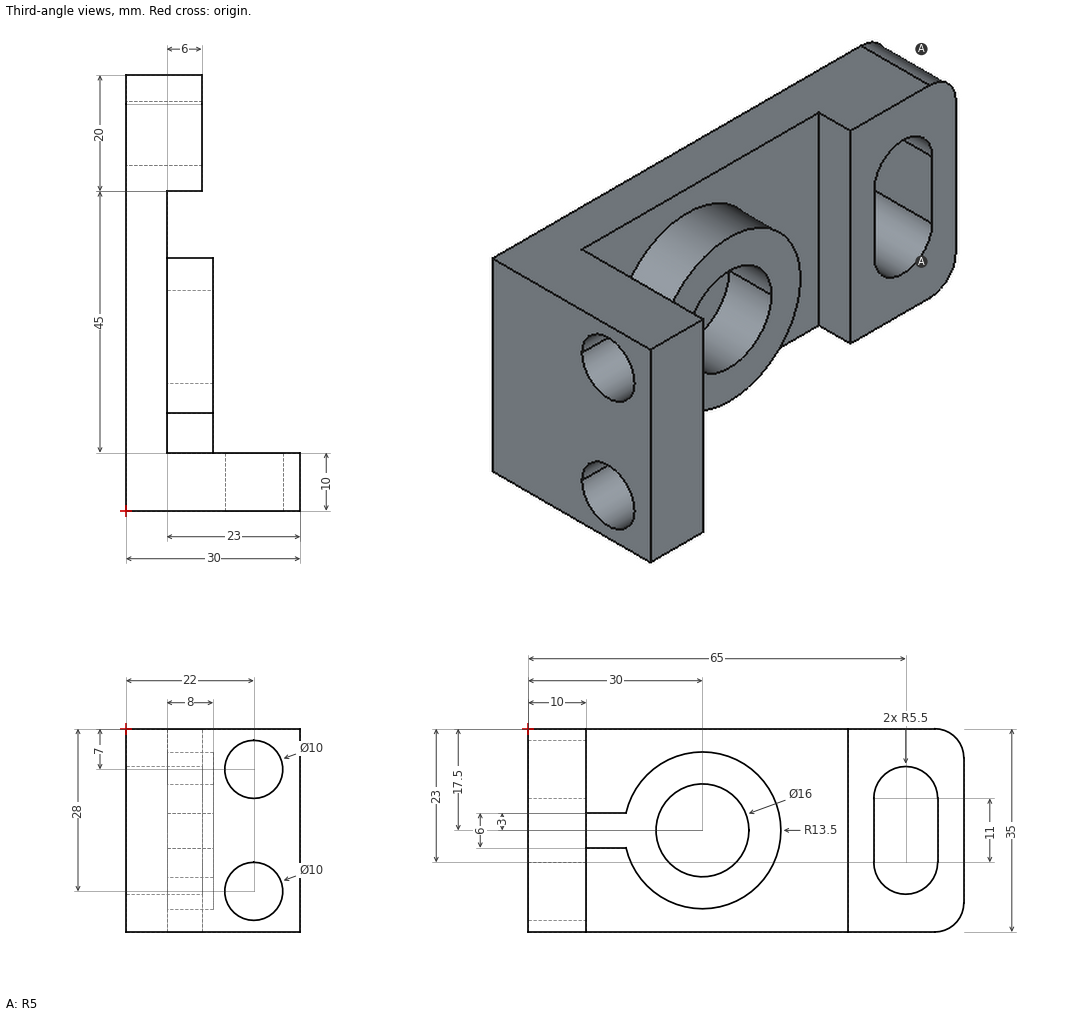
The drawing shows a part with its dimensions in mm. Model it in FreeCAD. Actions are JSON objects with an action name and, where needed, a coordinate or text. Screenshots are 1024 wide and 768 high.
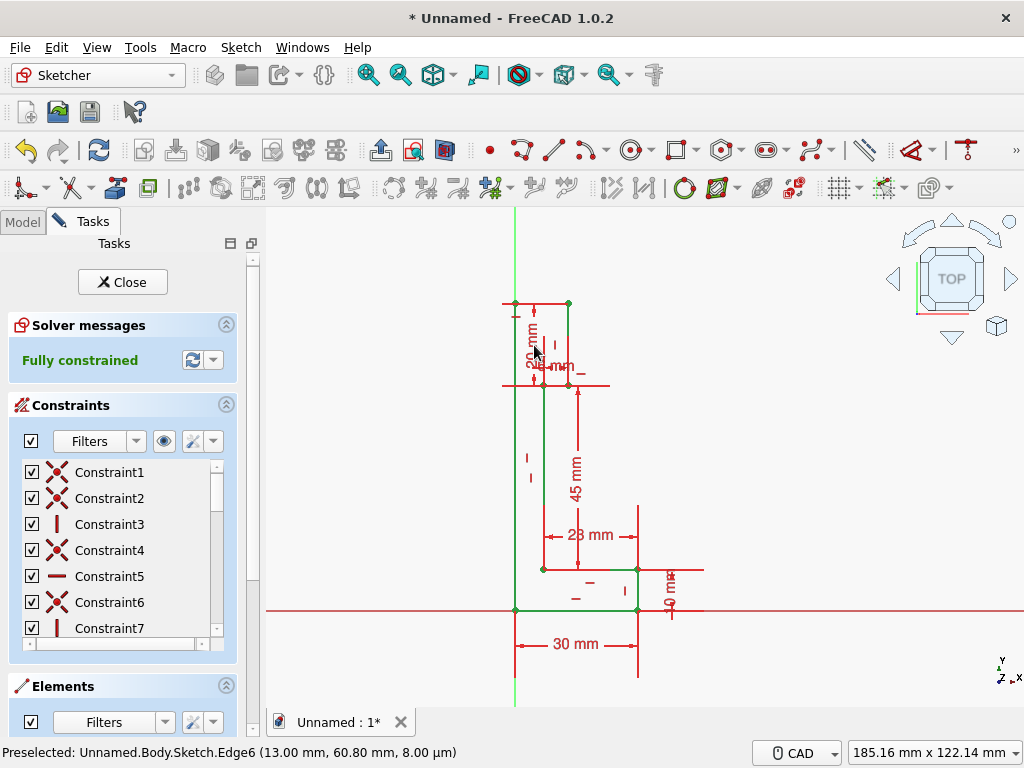
{"action": "left_click", "coordinate": [123, 282]}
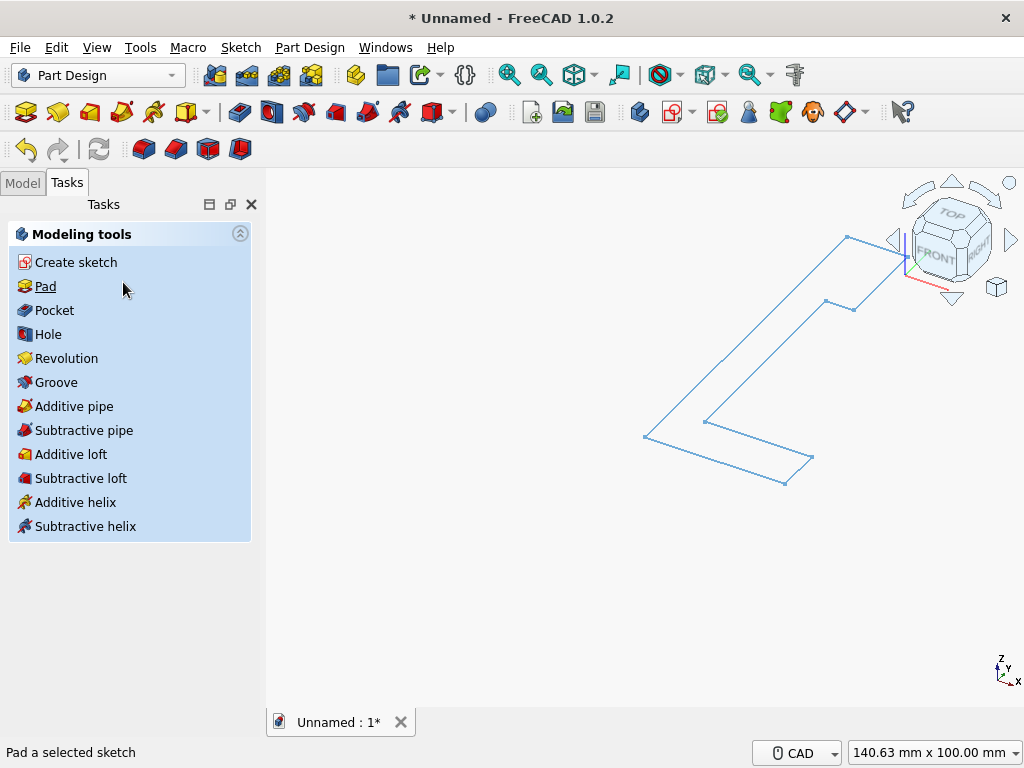
{"action": "left_click", "coordinate": [26, 112]}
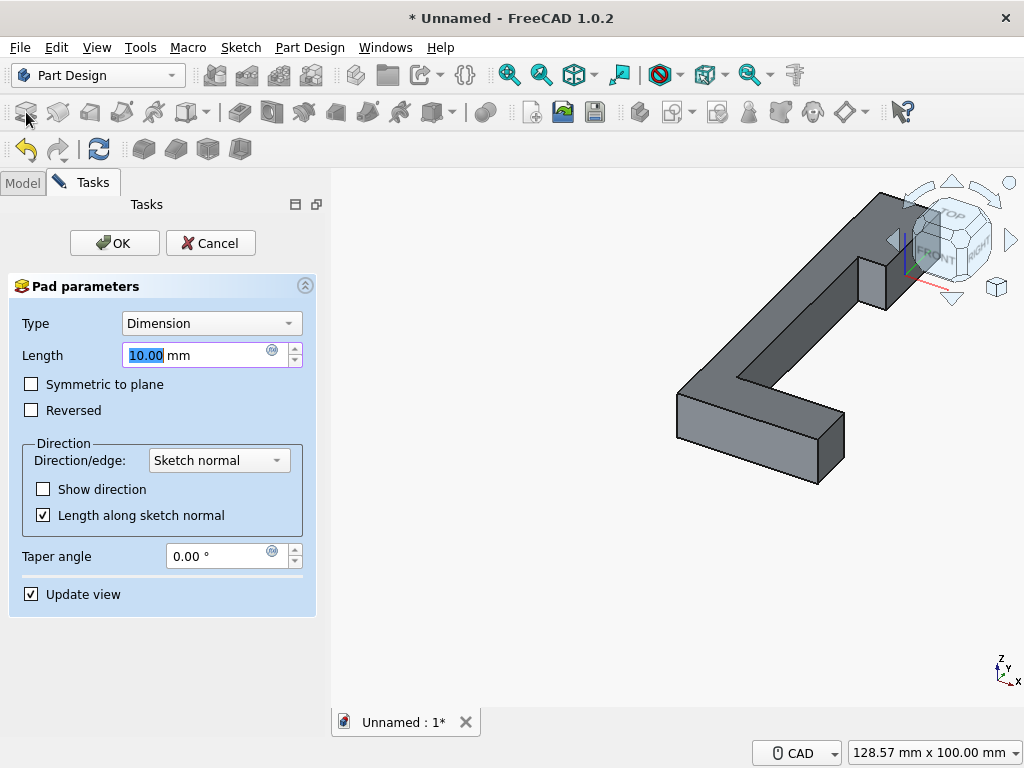
{"action": "type", "text": "35"}
{"action": "key", "text": "Tab"}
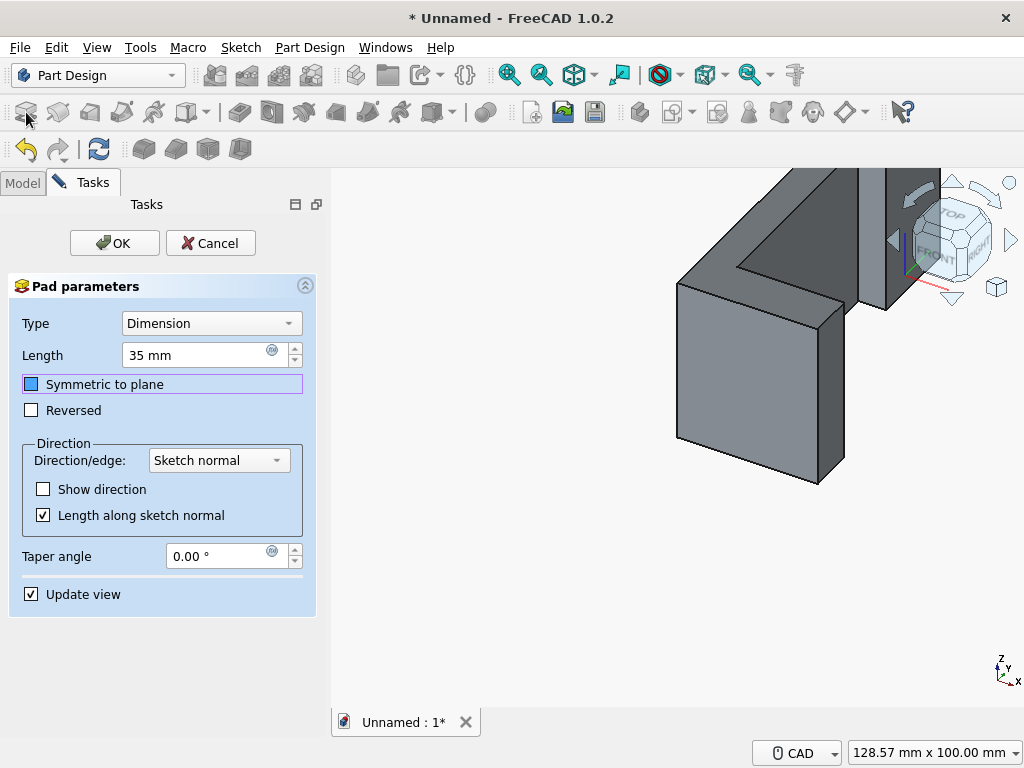
{"action": "left_click", "coordinate": [30, 410]}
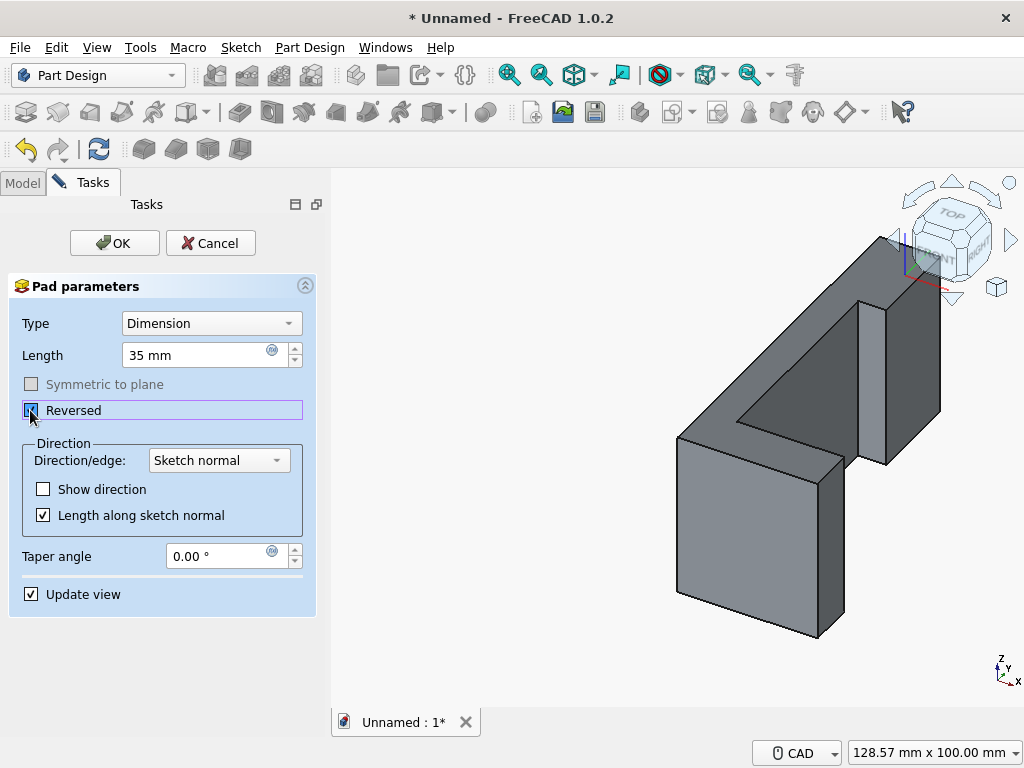
{"action": "left_click", "coordinate": [115, 243]}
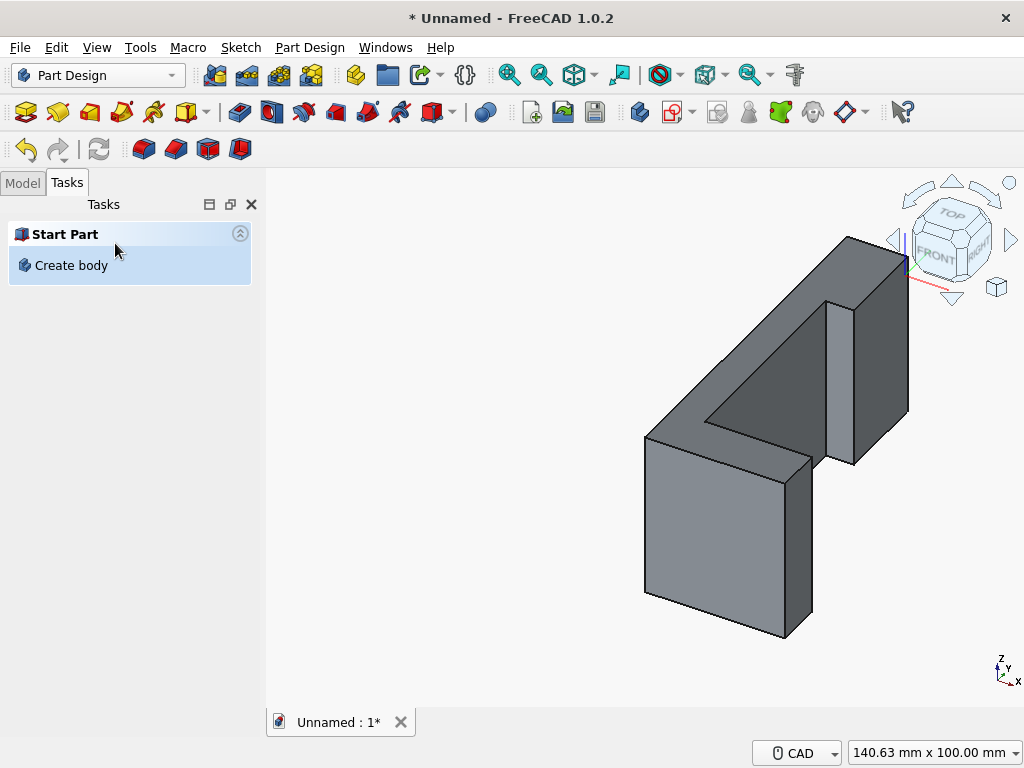
{"action": "key", "text": "4"}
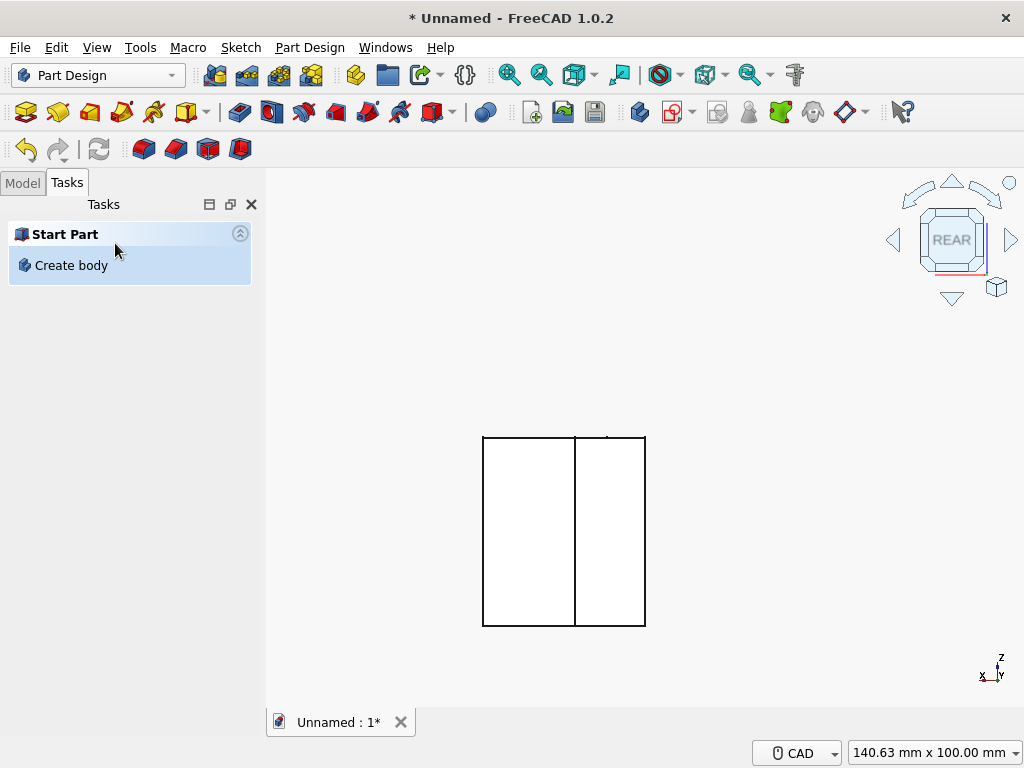
{"action": "left_click", "coordinate": [510, 76]}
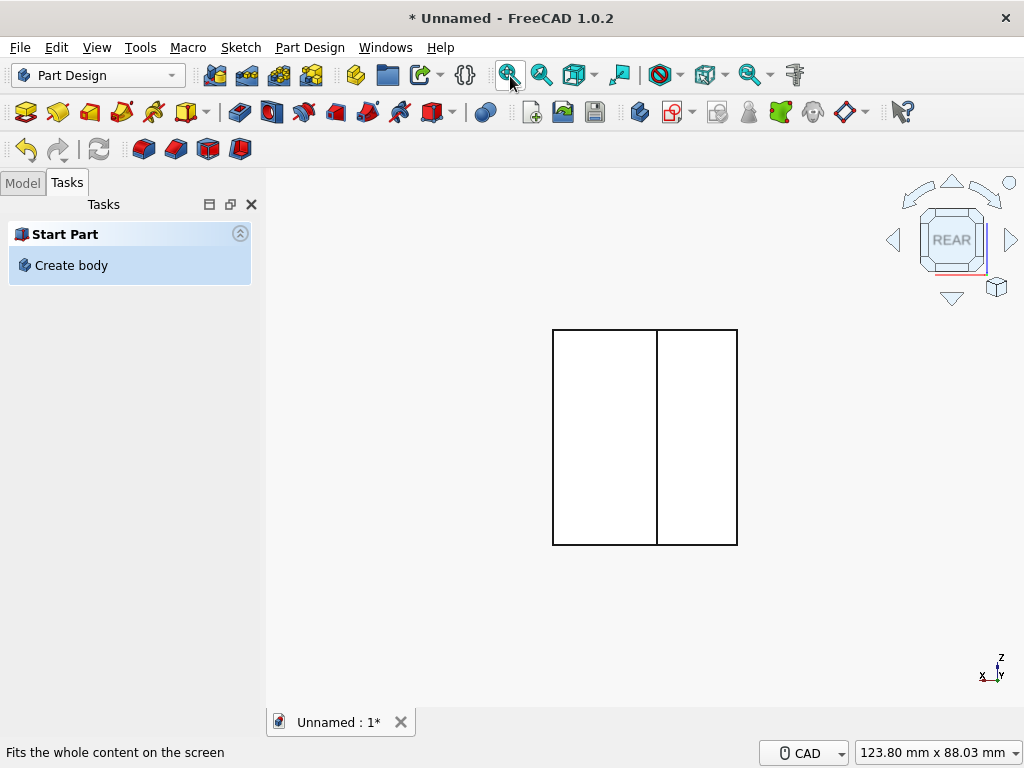
{"action": "left_click", "coordinate": [624, 406]}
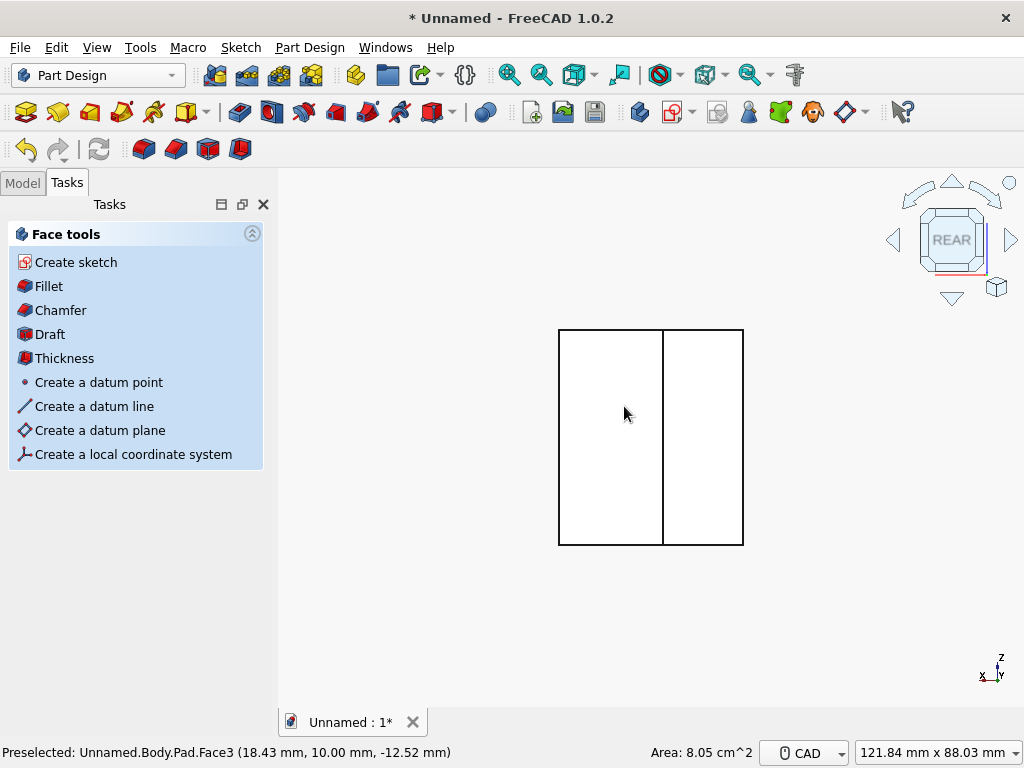
{"action": "left_click", "coordinate": [672, 112]}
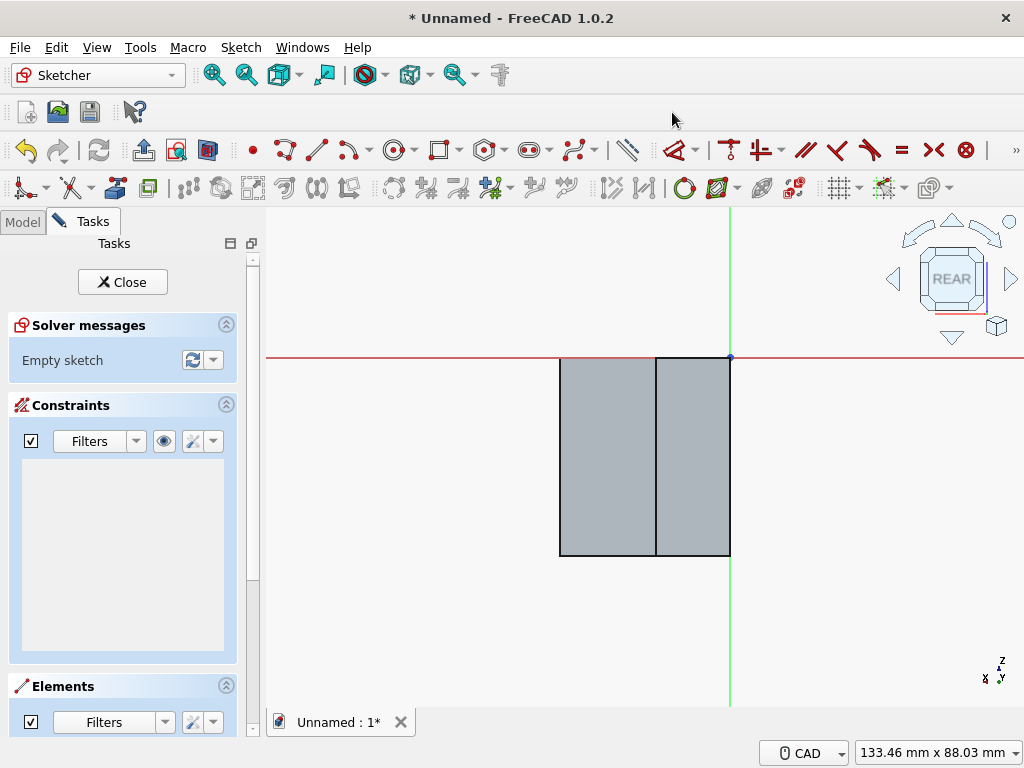
{"action": "left_click", "coordinate": [208, 150]}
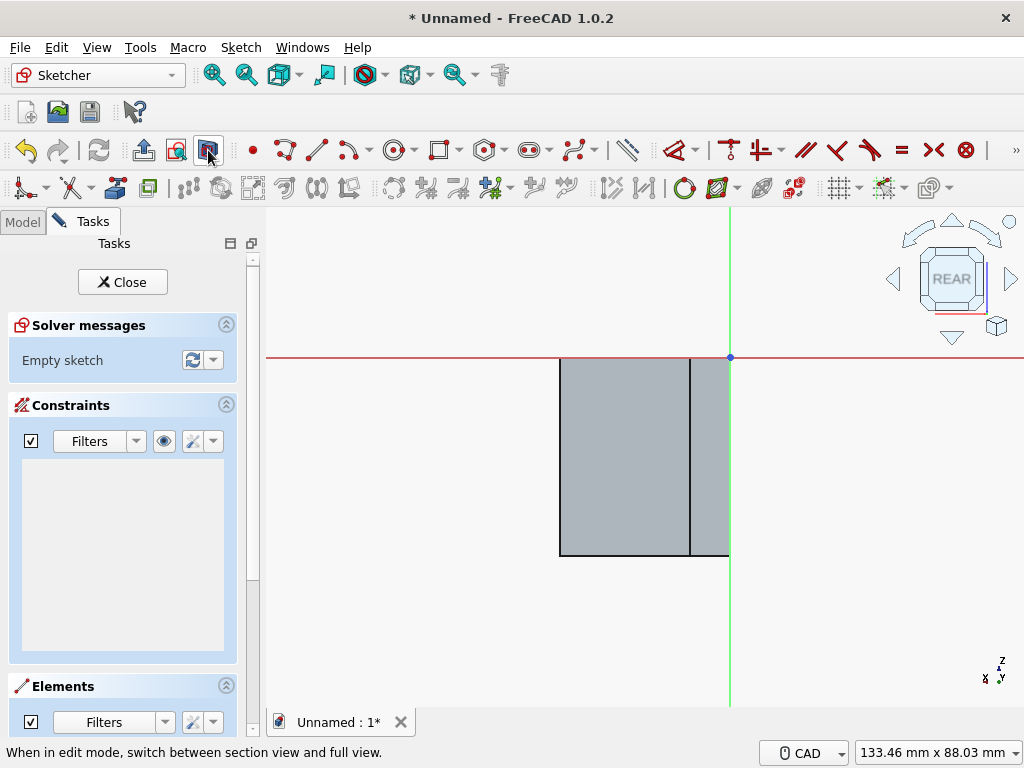
{"action": "scroll", "coordinate": [611, 528], "scroll_direction": "up", "scroll_amount": 9}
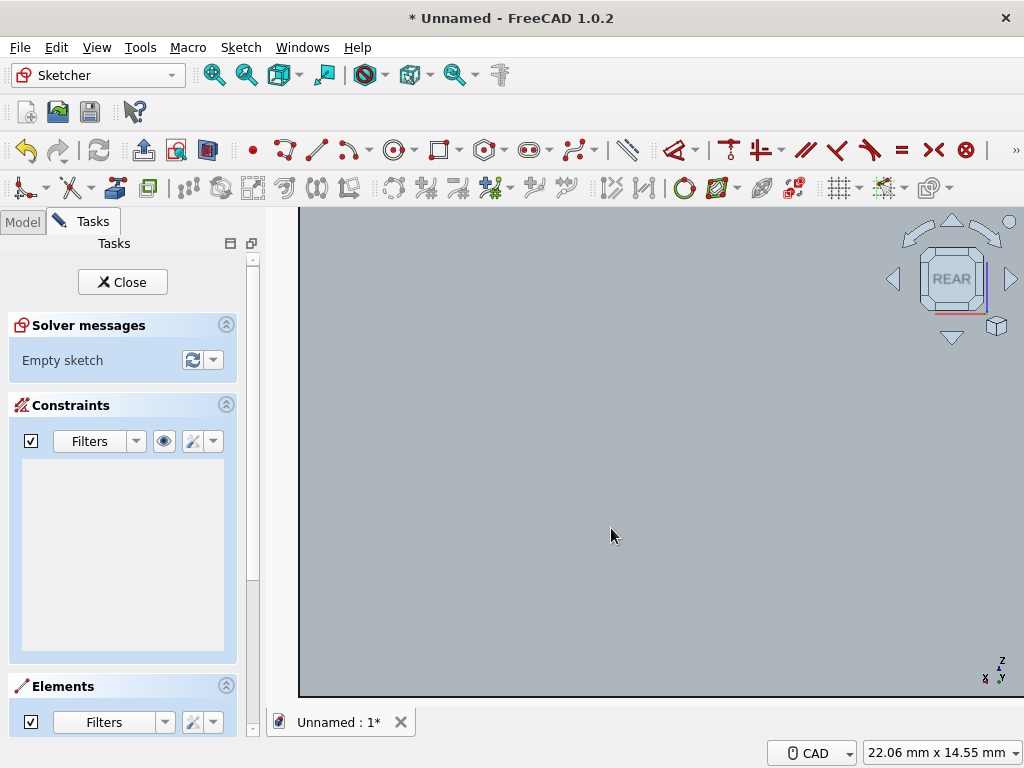
{"action": "left_click", "coordinate": [394, 150]}